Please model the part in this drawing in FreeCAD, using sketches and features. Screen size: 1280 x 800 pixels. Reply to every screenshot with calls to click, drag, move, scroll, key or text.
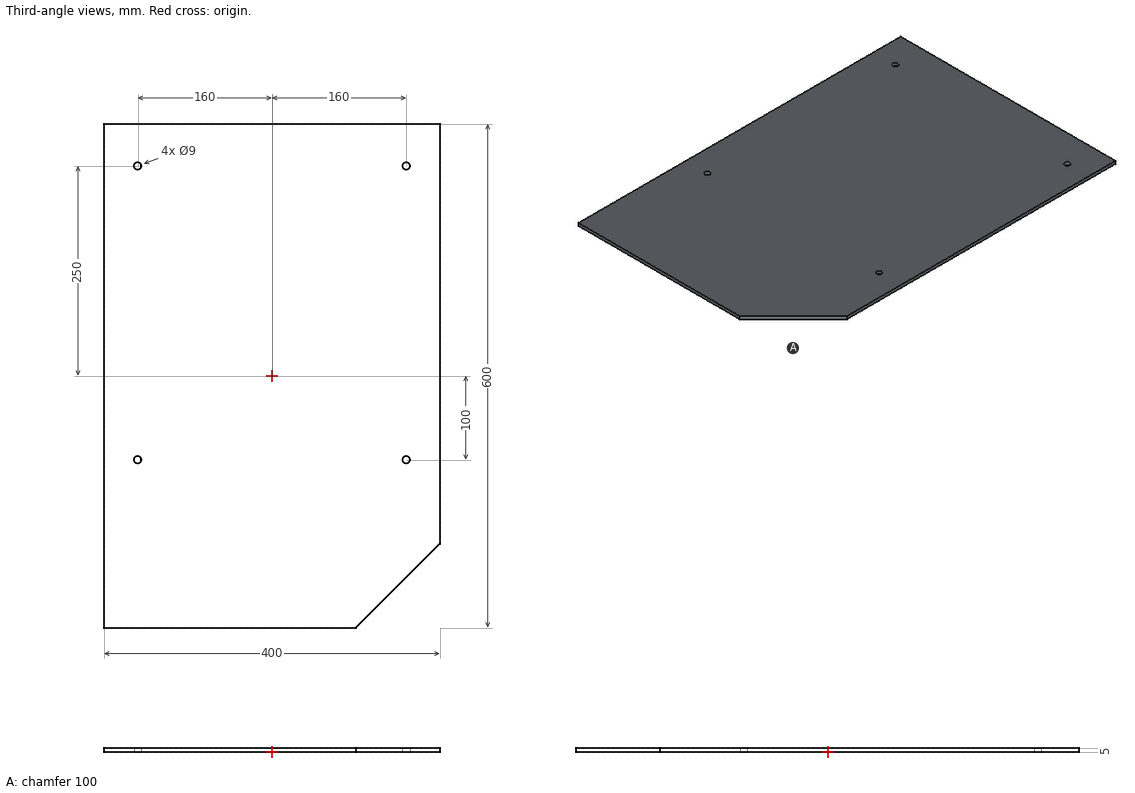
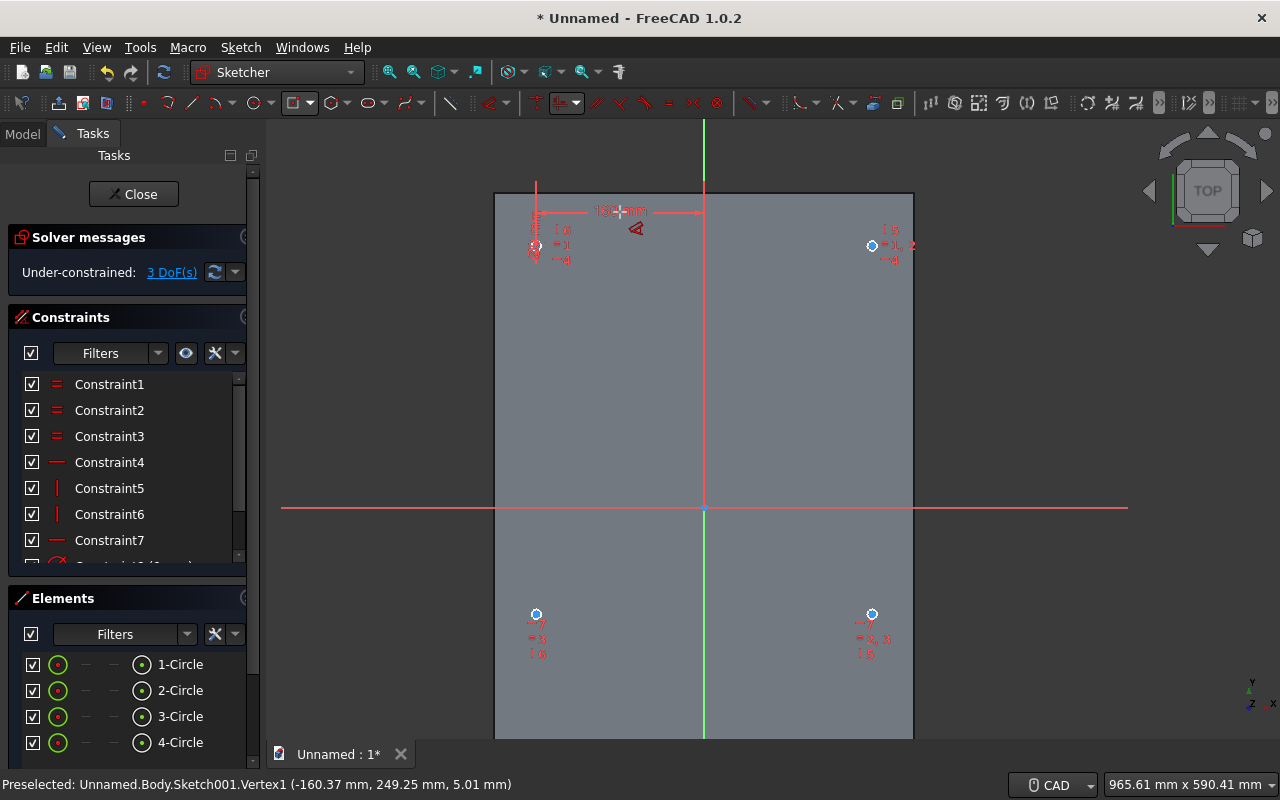
click(536, 246)
click(502, 377)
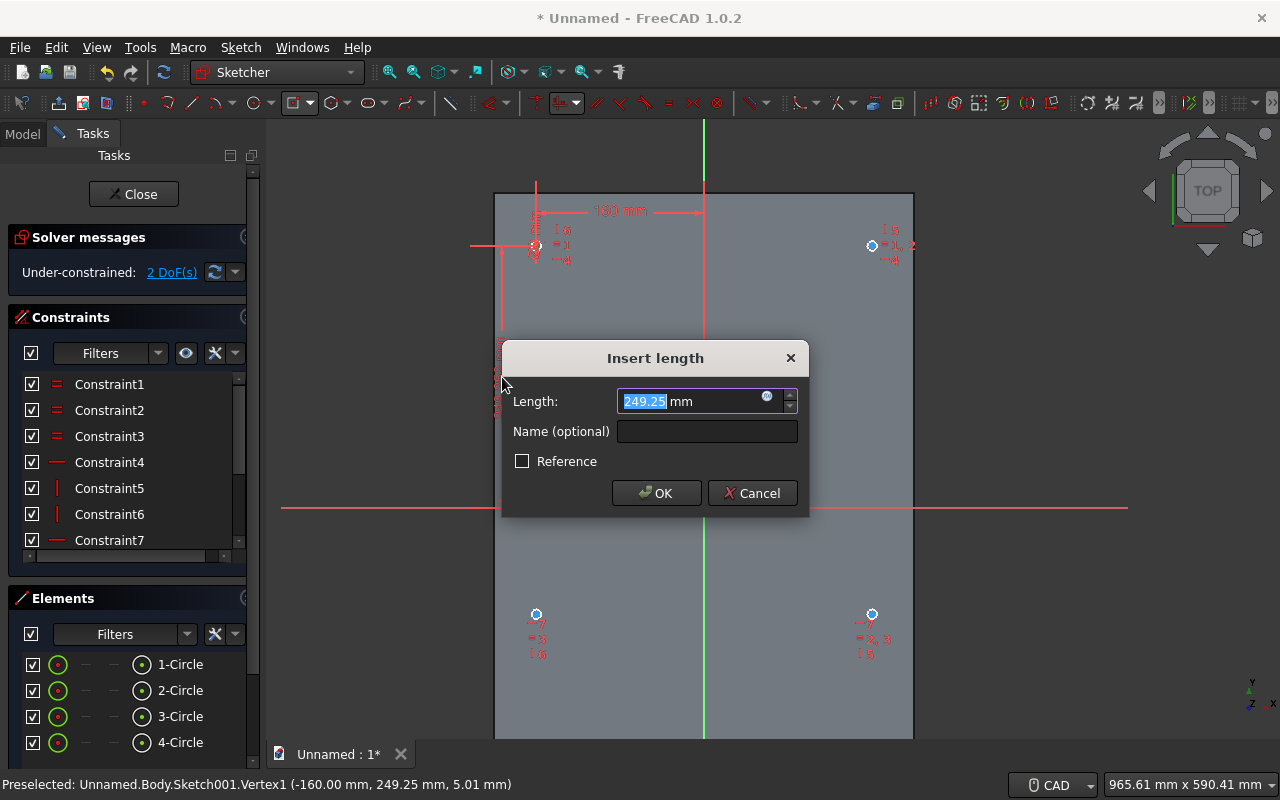
text(250)
key(Return)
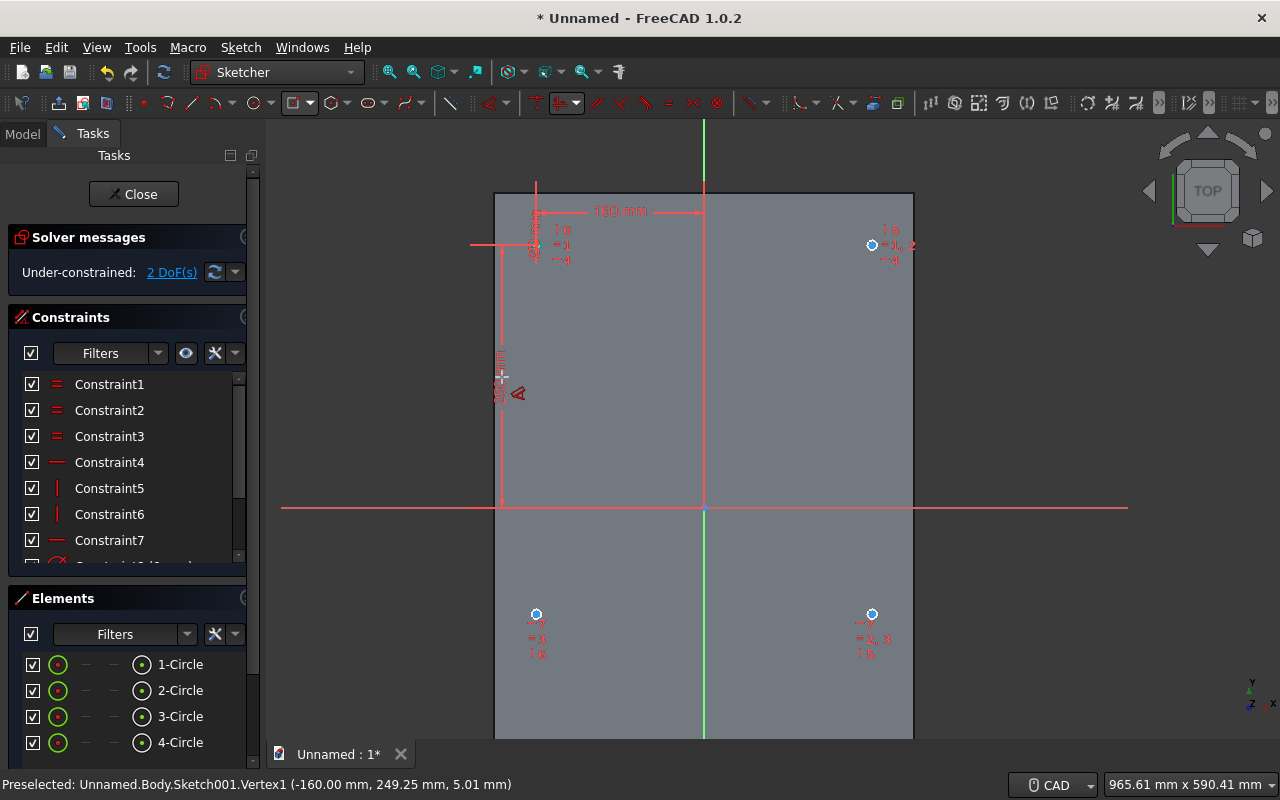
click(872, 245)
click(788, 211)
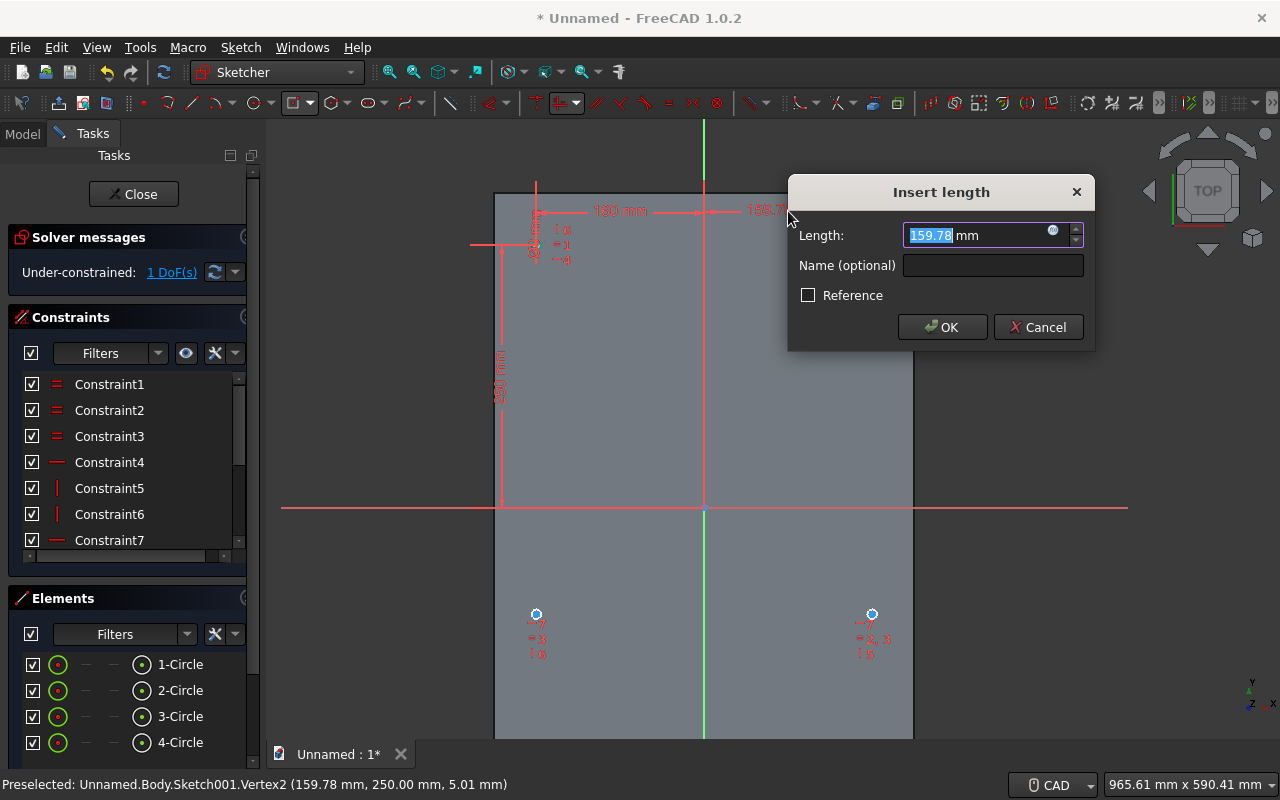
text(160)
key(Return)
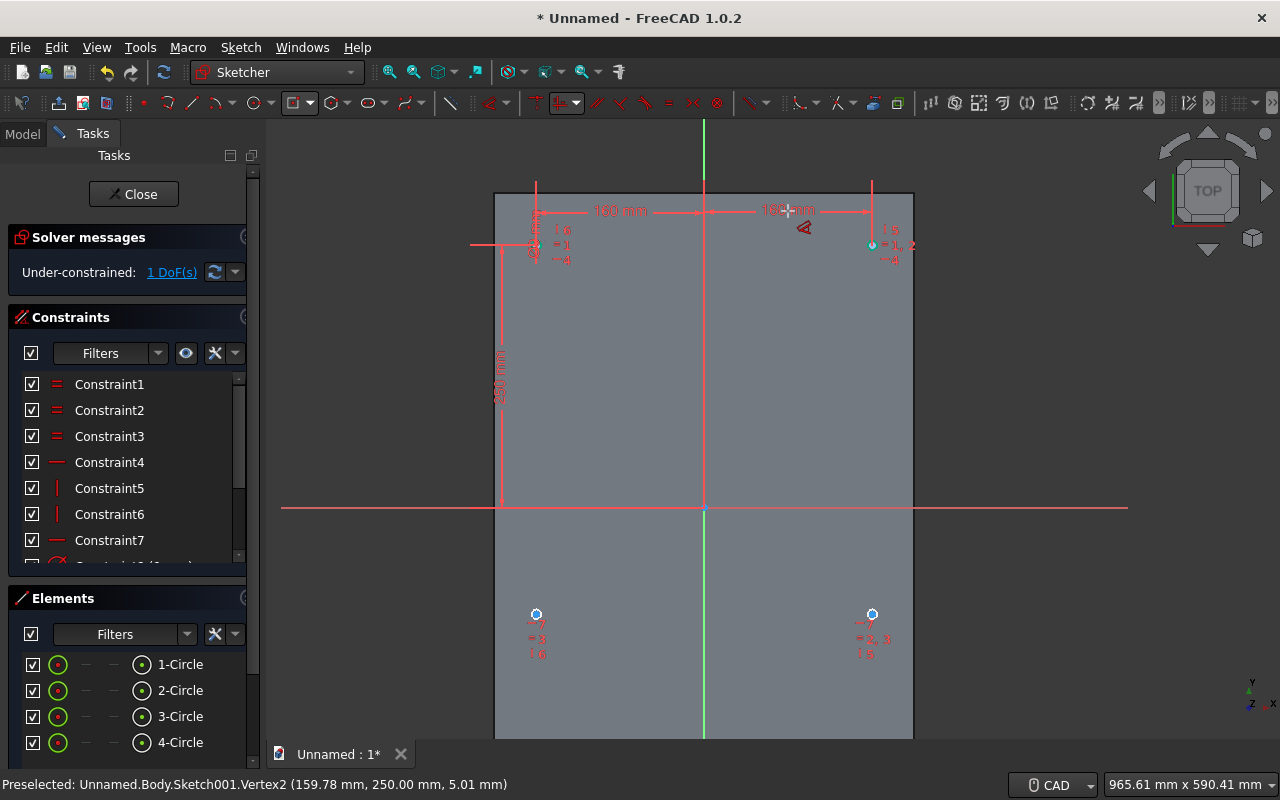
click(872, 614)
click(906, 561)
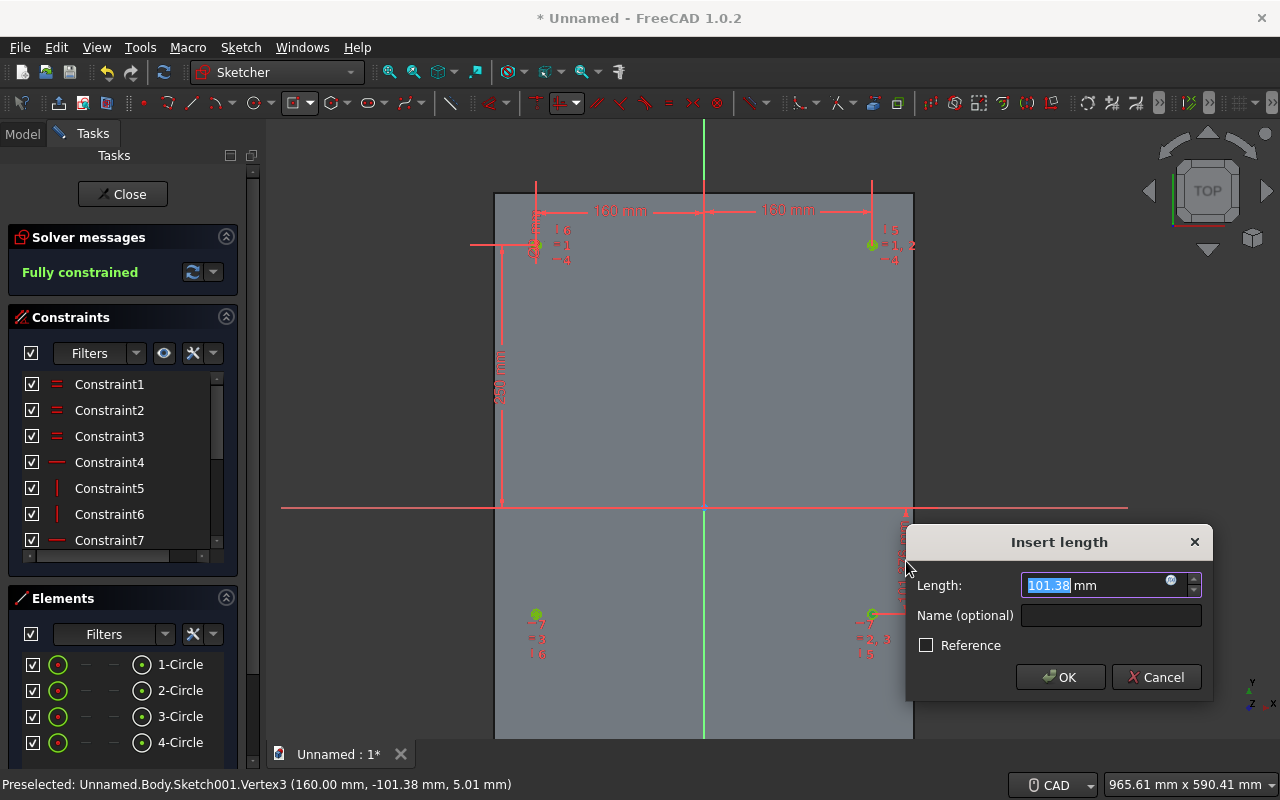
text(100)
key(Return)
key(Escape)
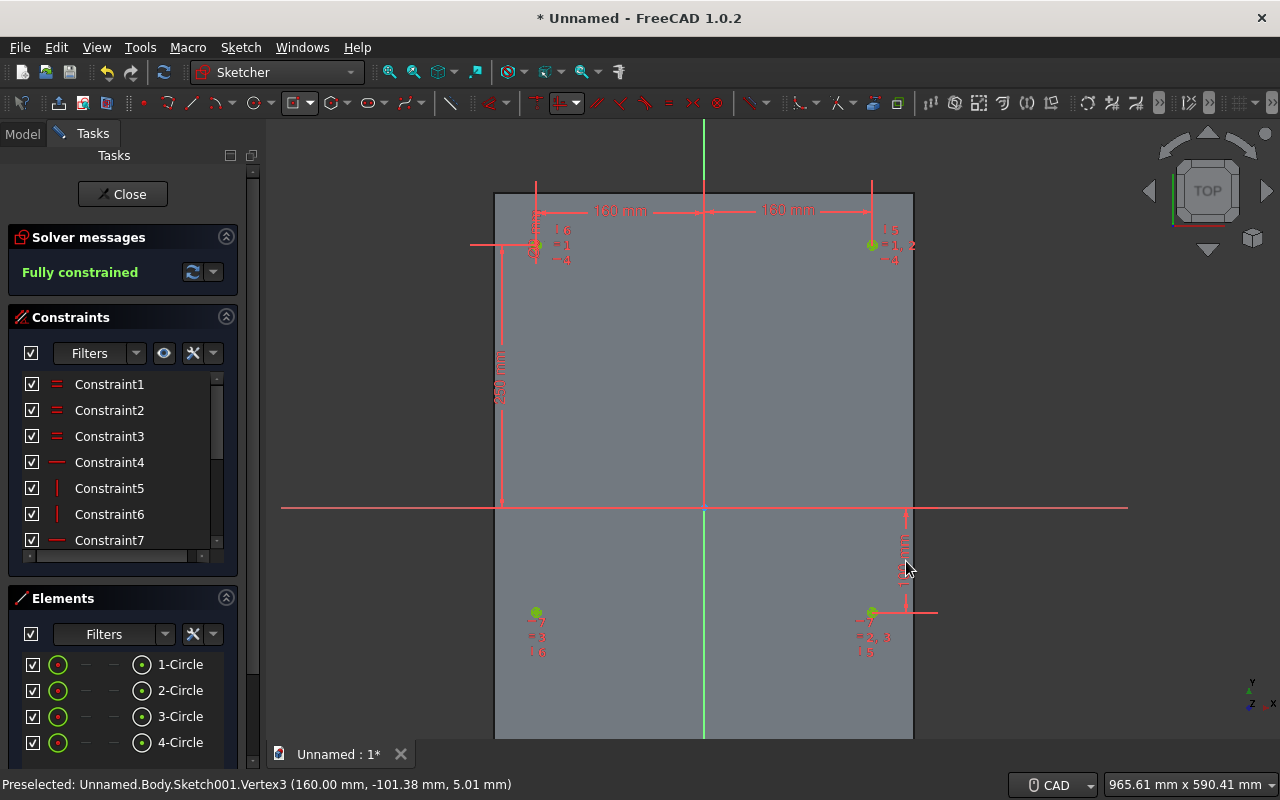
click(123, 194)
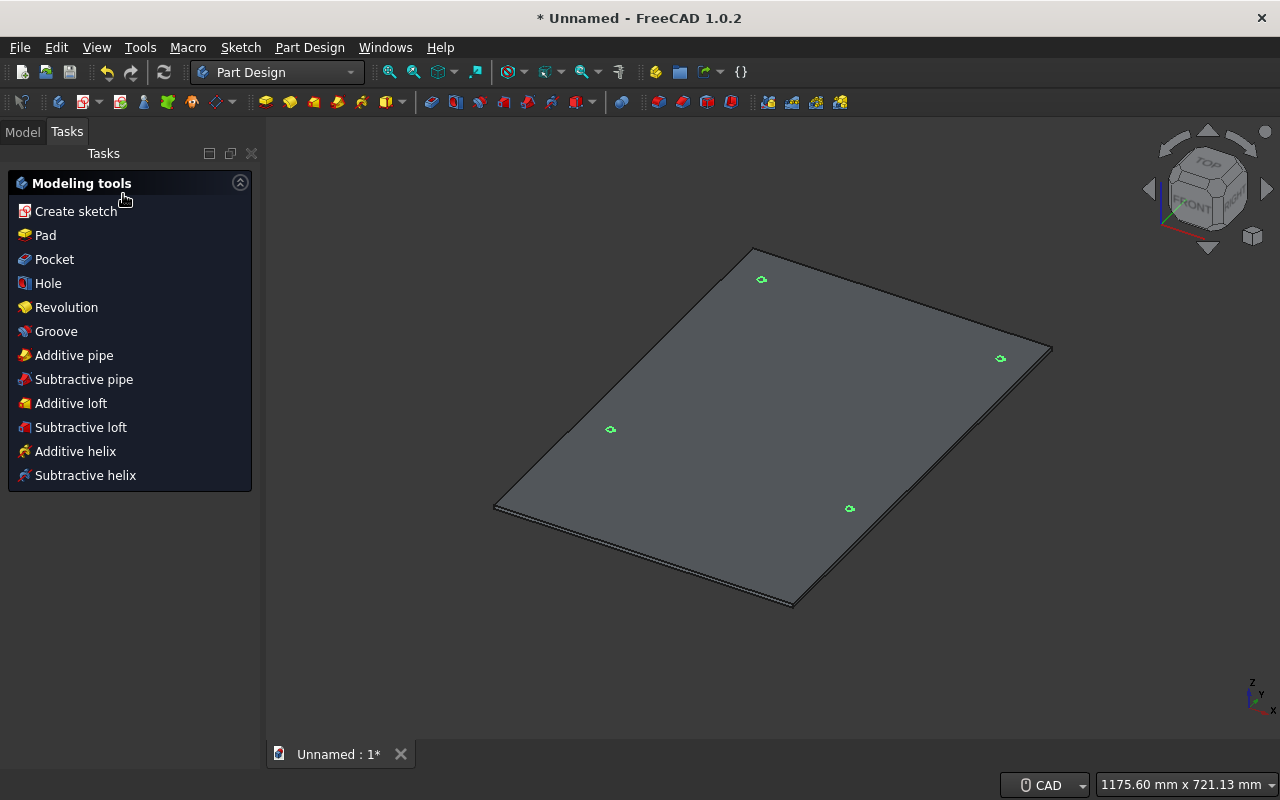
click(432, 102)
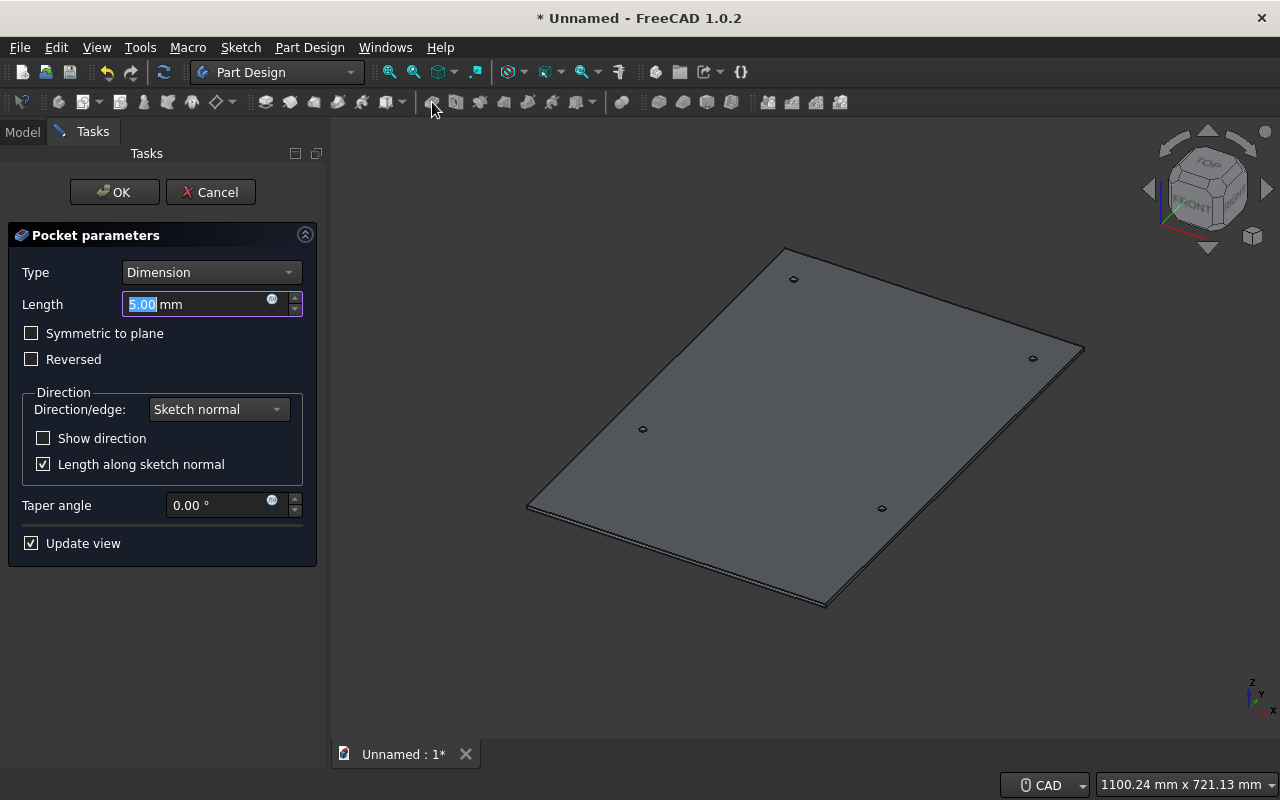
click(212, 272)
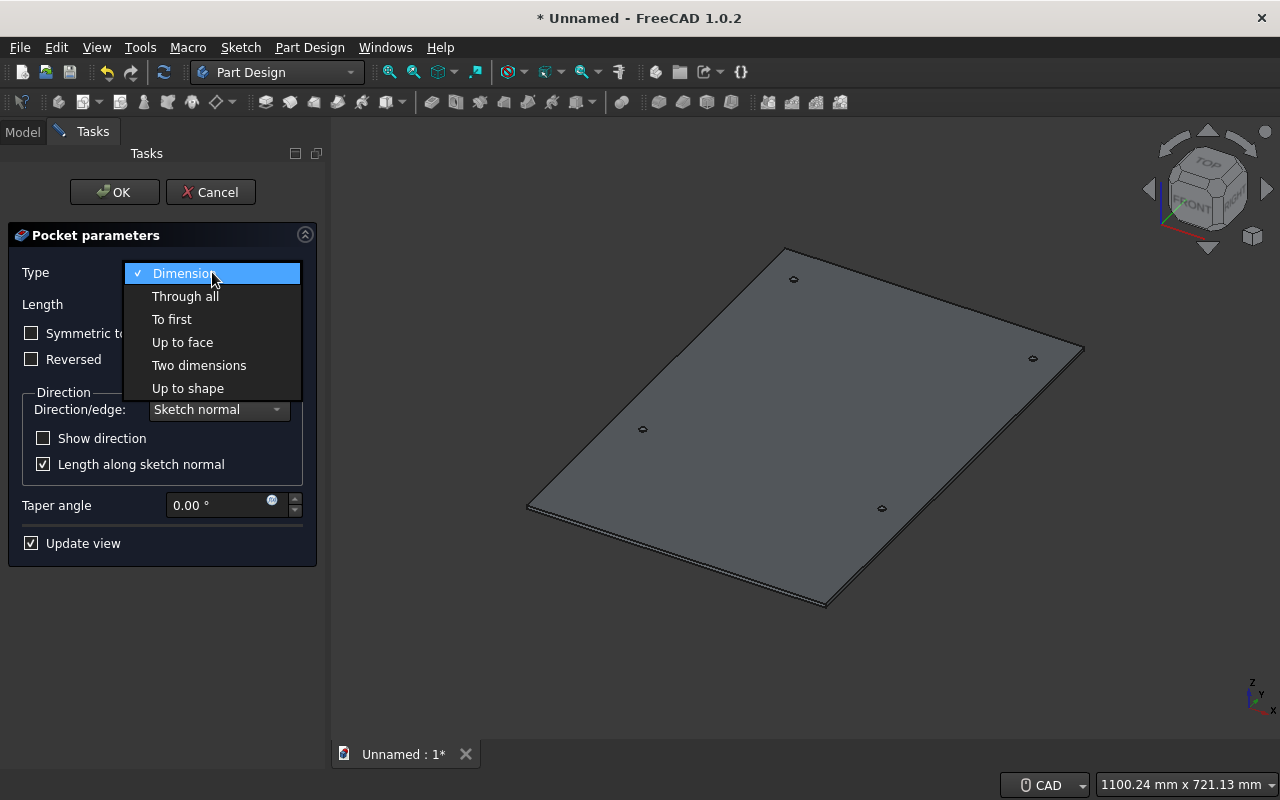
click(212, 296)